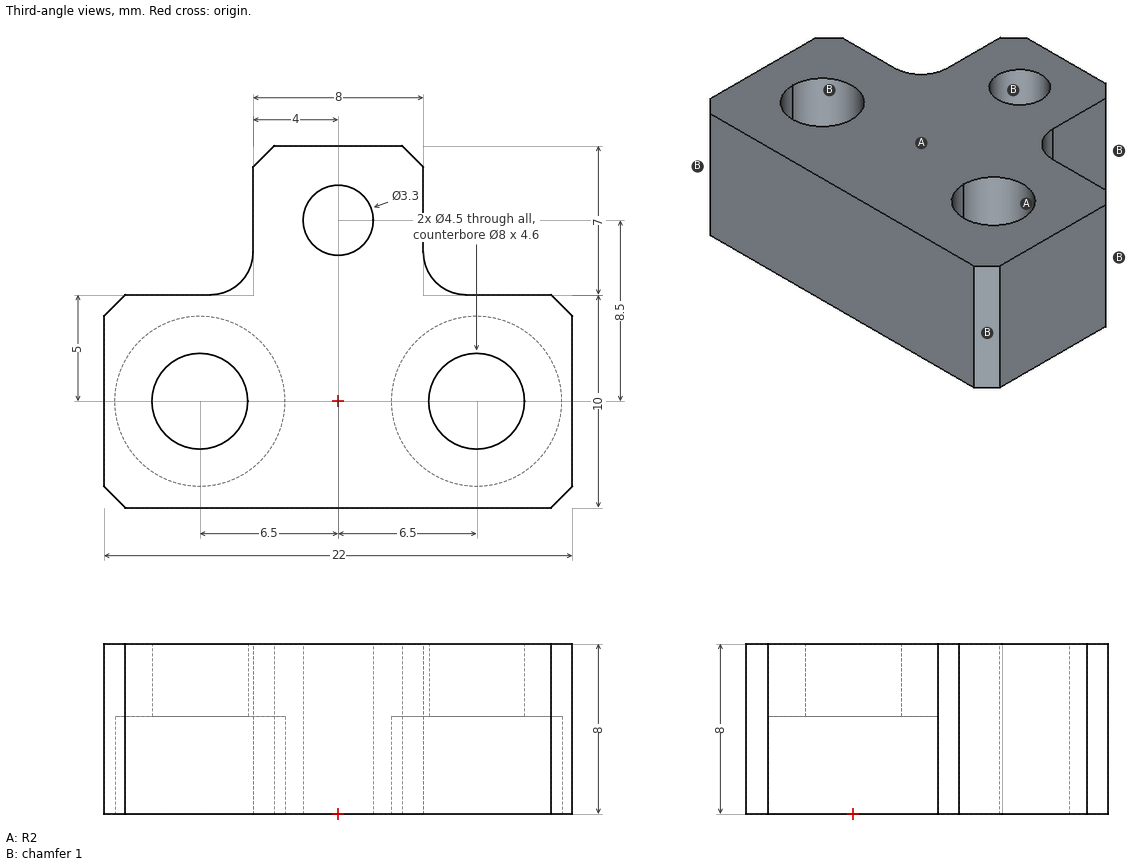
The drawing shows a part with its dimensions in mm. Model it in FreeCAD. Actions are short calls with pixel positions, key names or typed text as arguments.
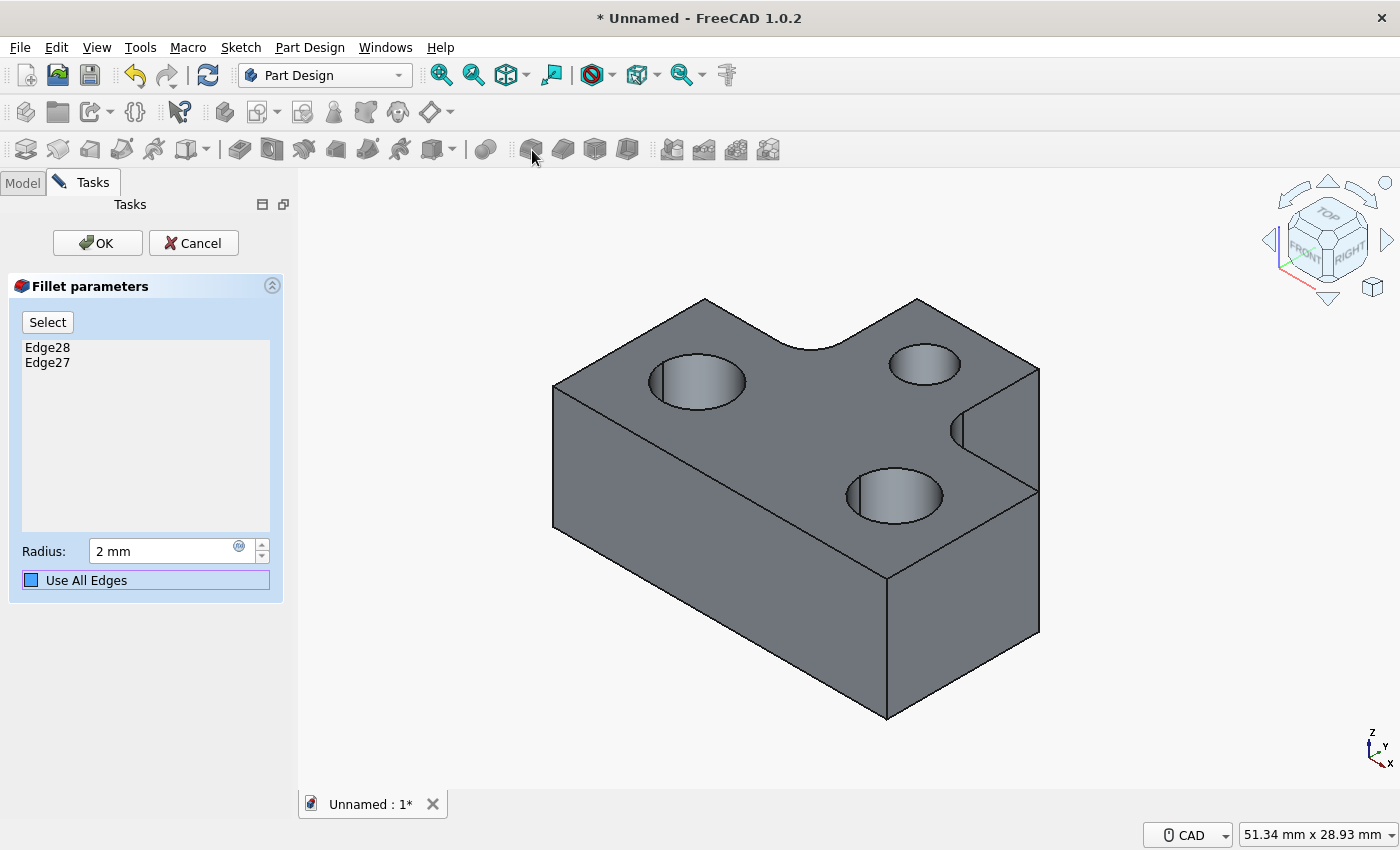
click(98, 243)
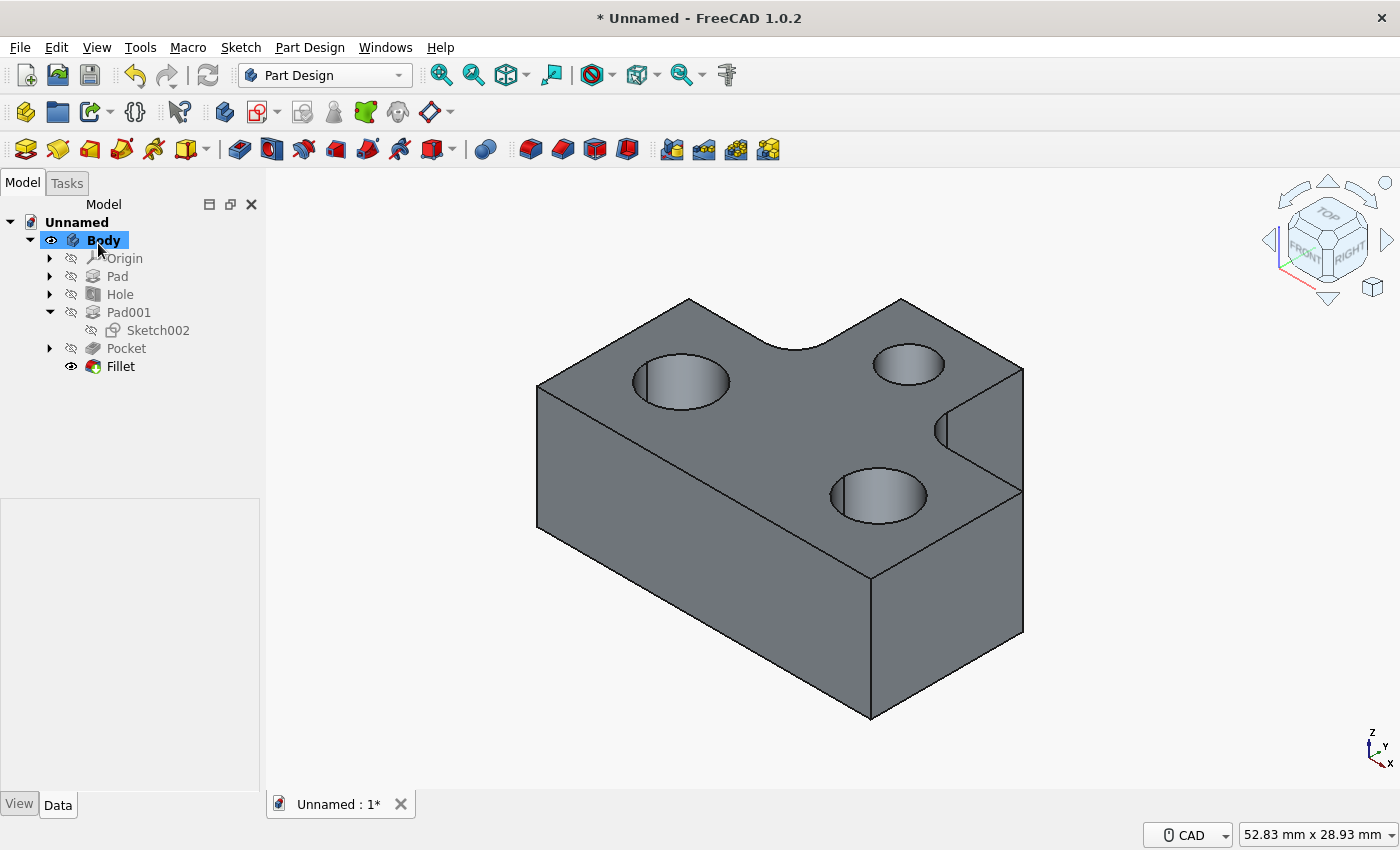
click(871, 648)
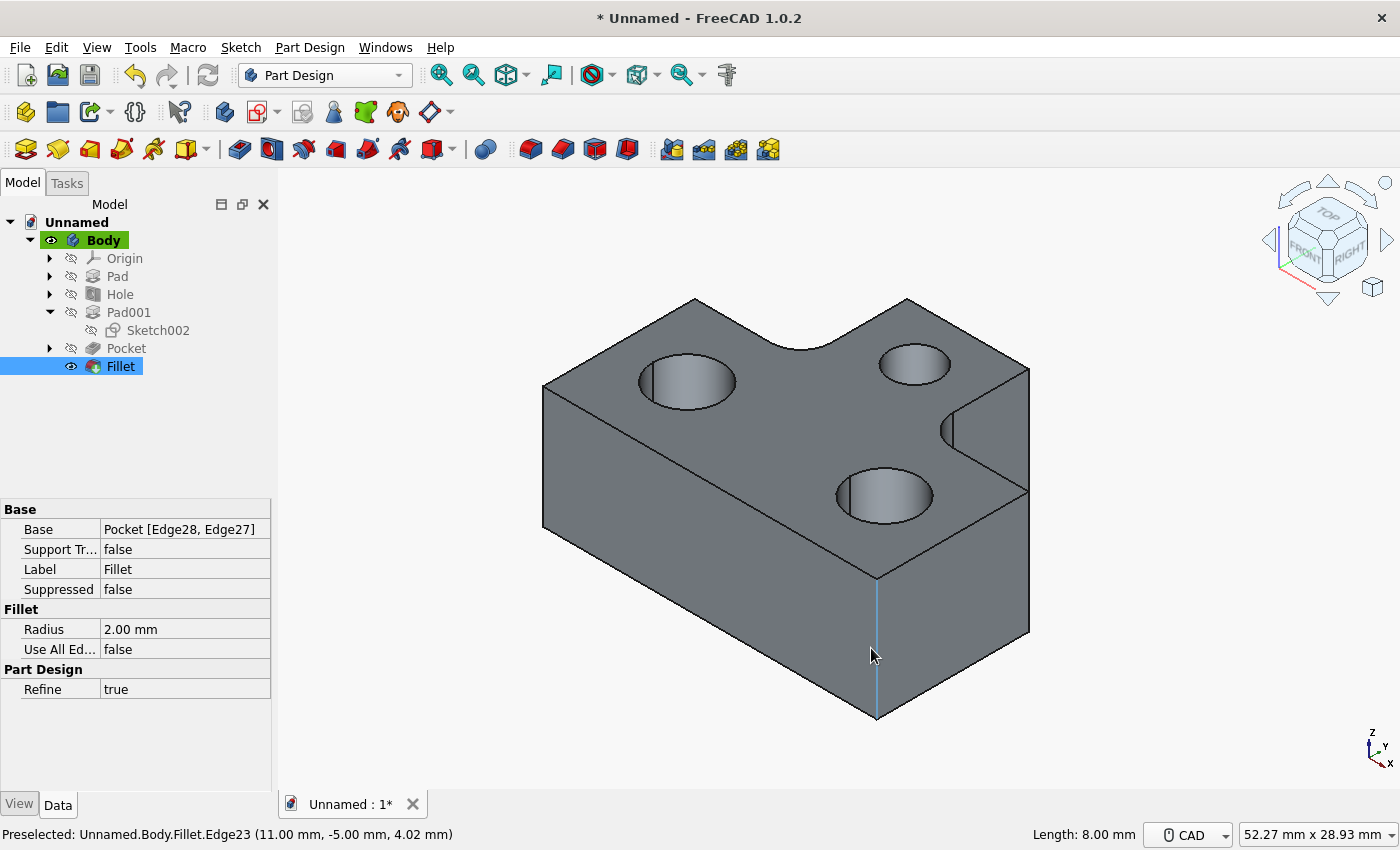
key(2)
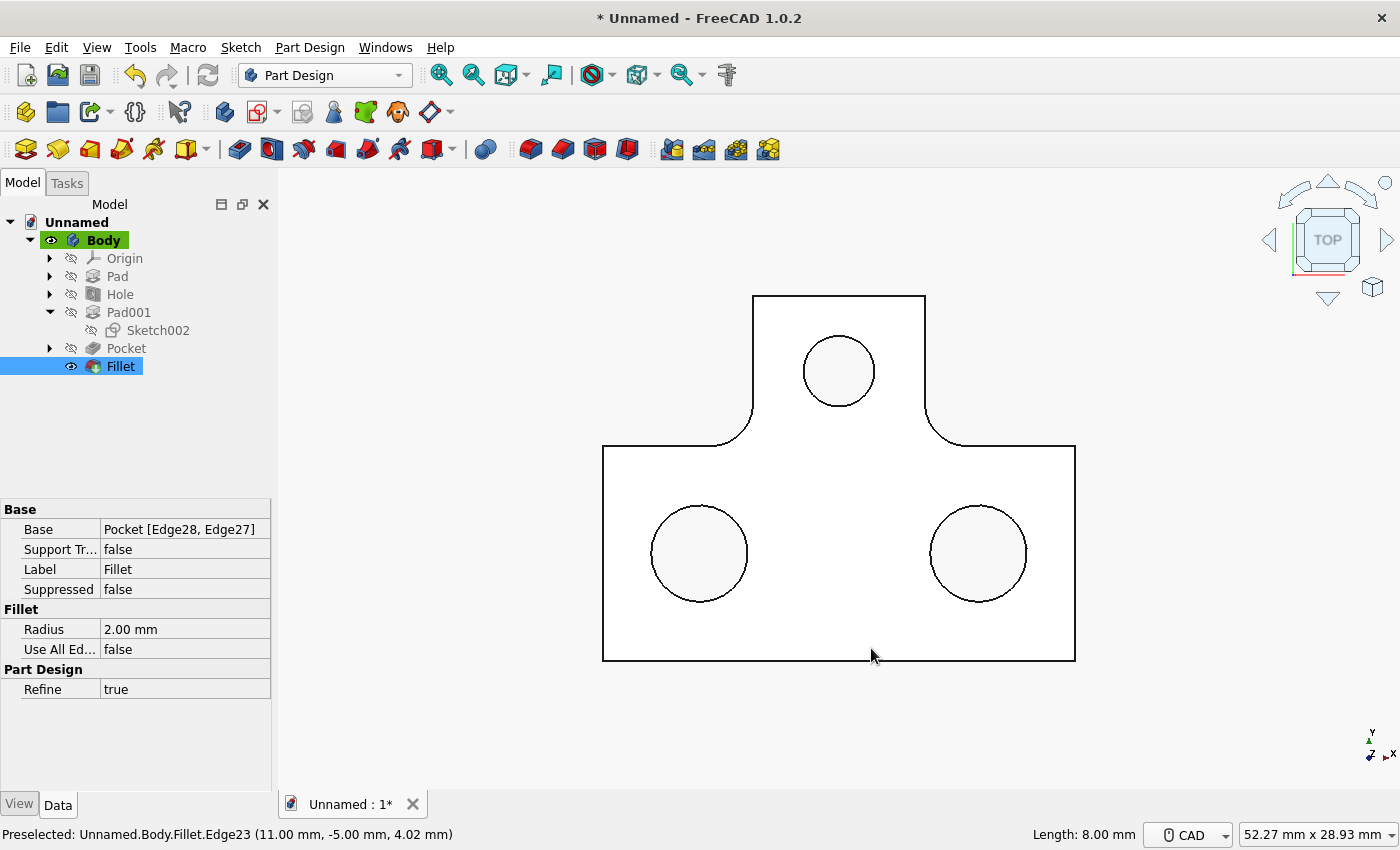
key(0)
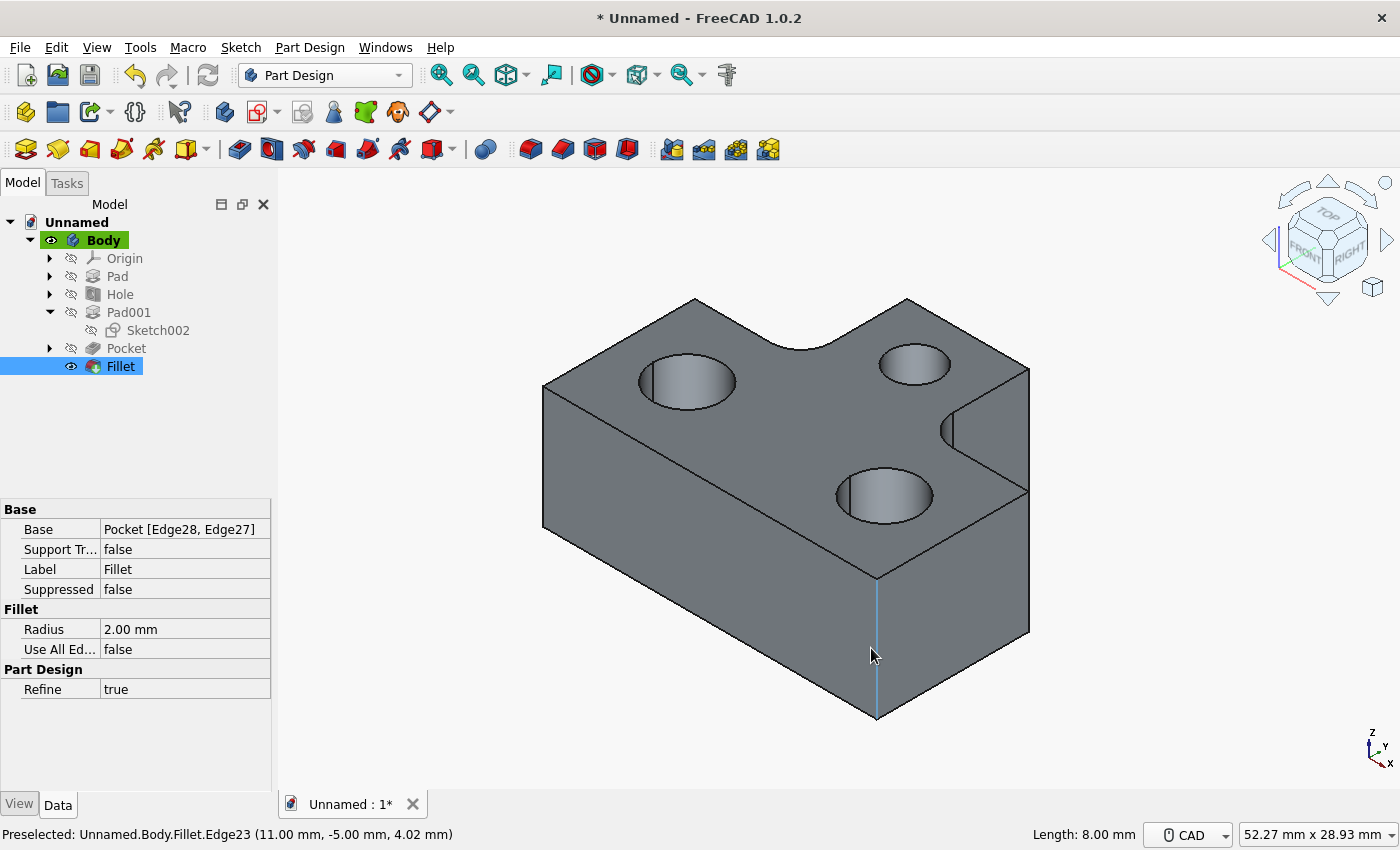
key(1)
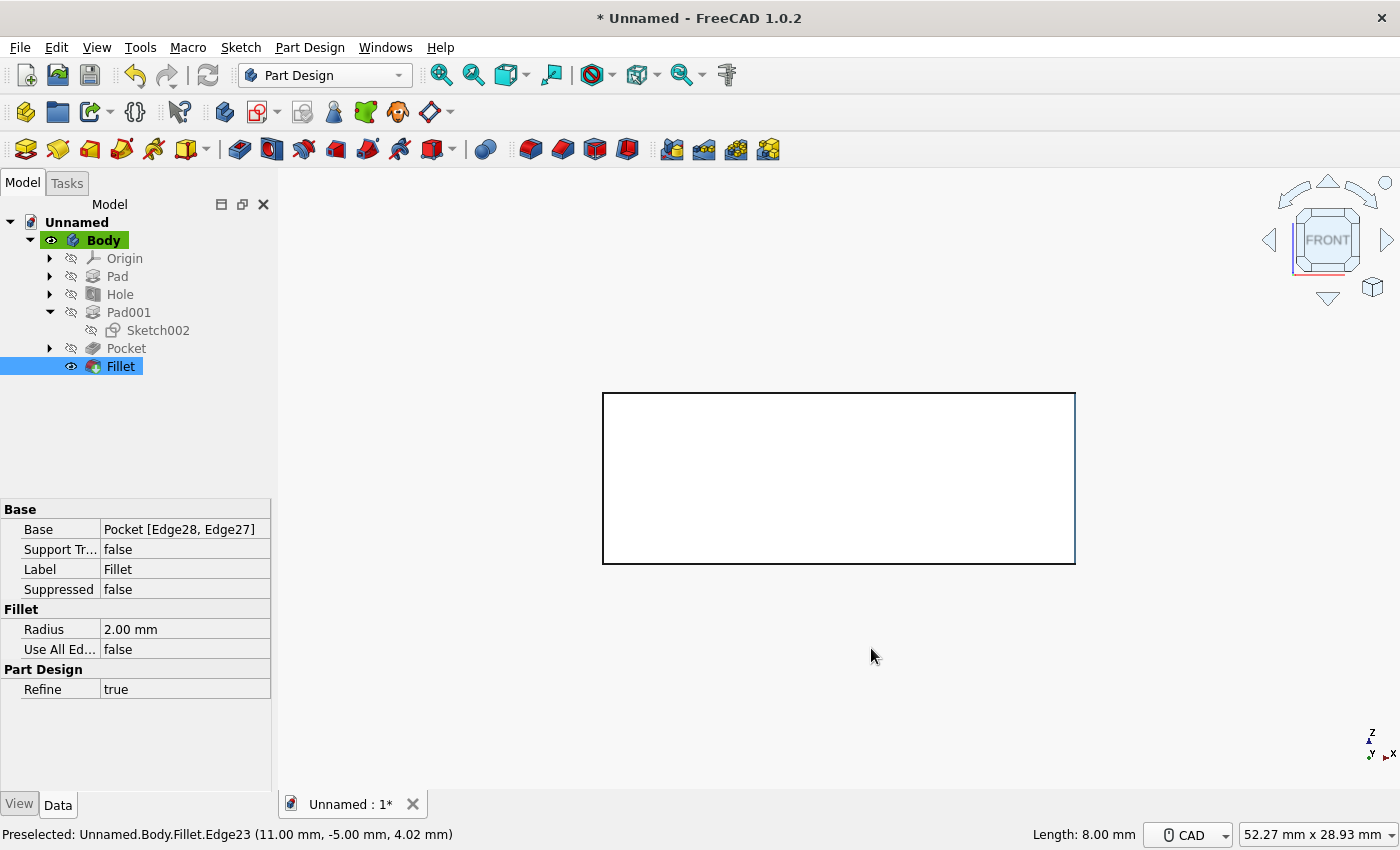
click(442, 76)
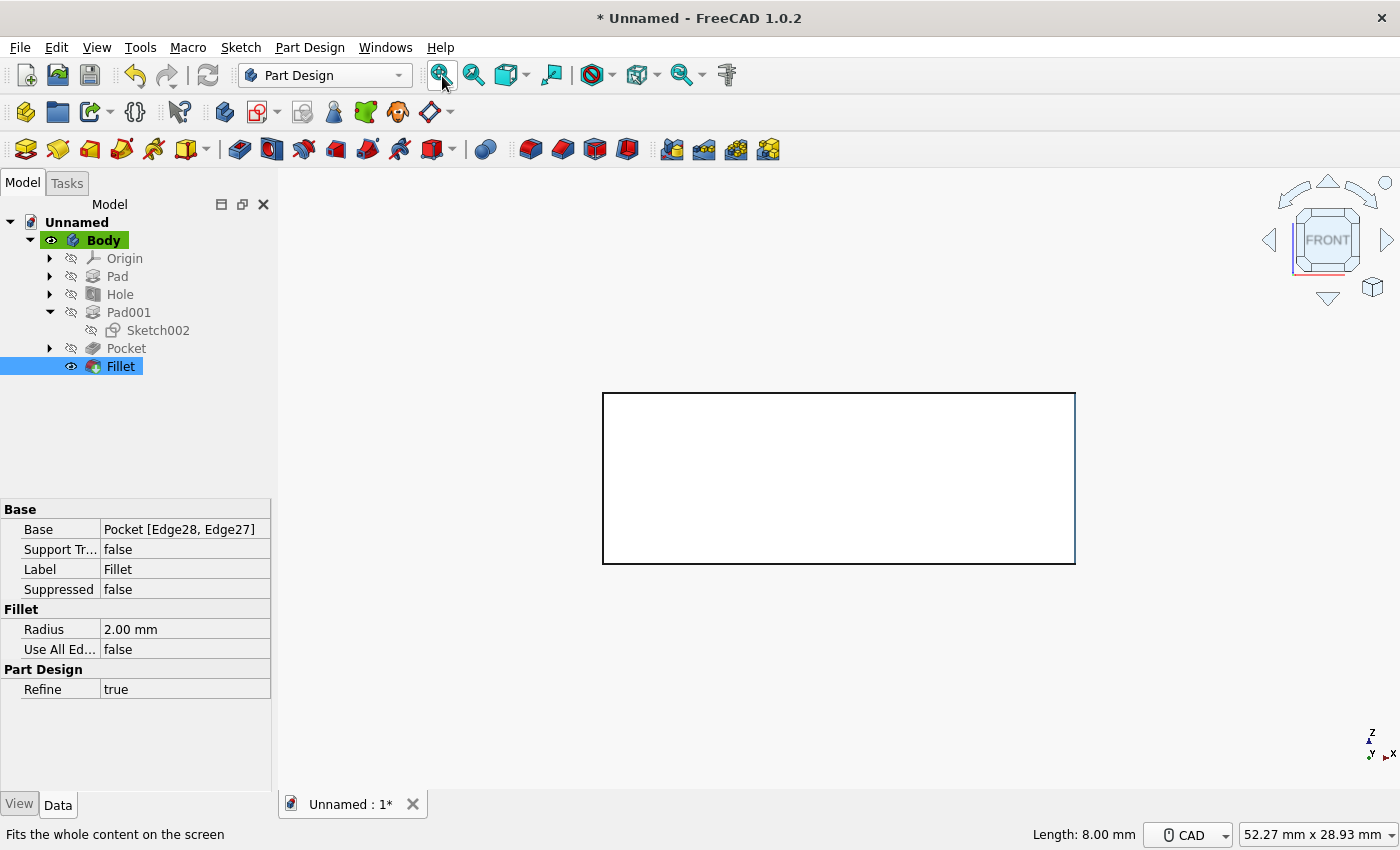
click(603, 478, ctrl)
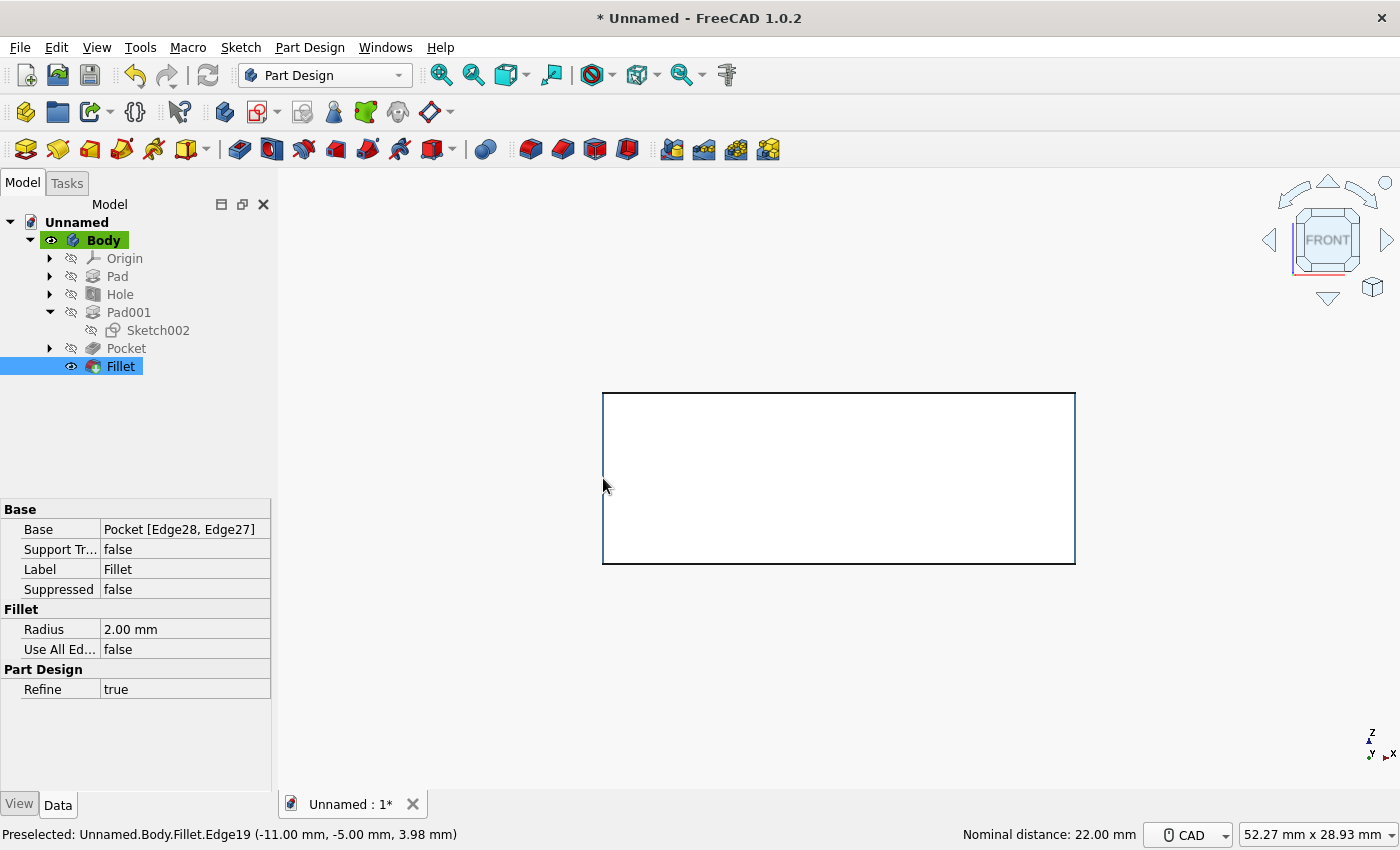
key(3)